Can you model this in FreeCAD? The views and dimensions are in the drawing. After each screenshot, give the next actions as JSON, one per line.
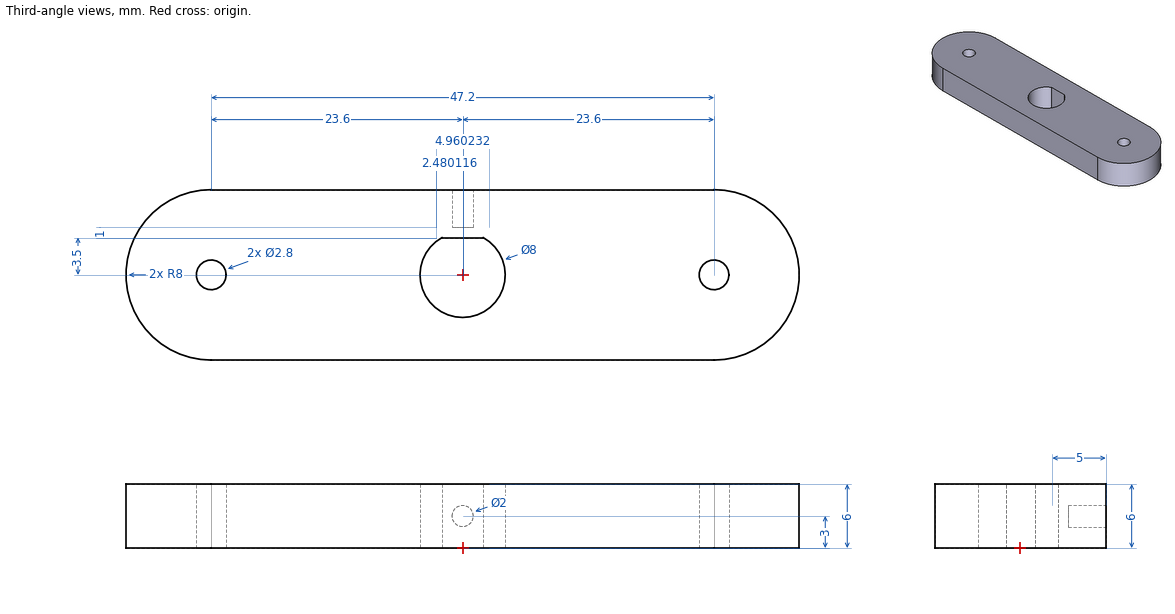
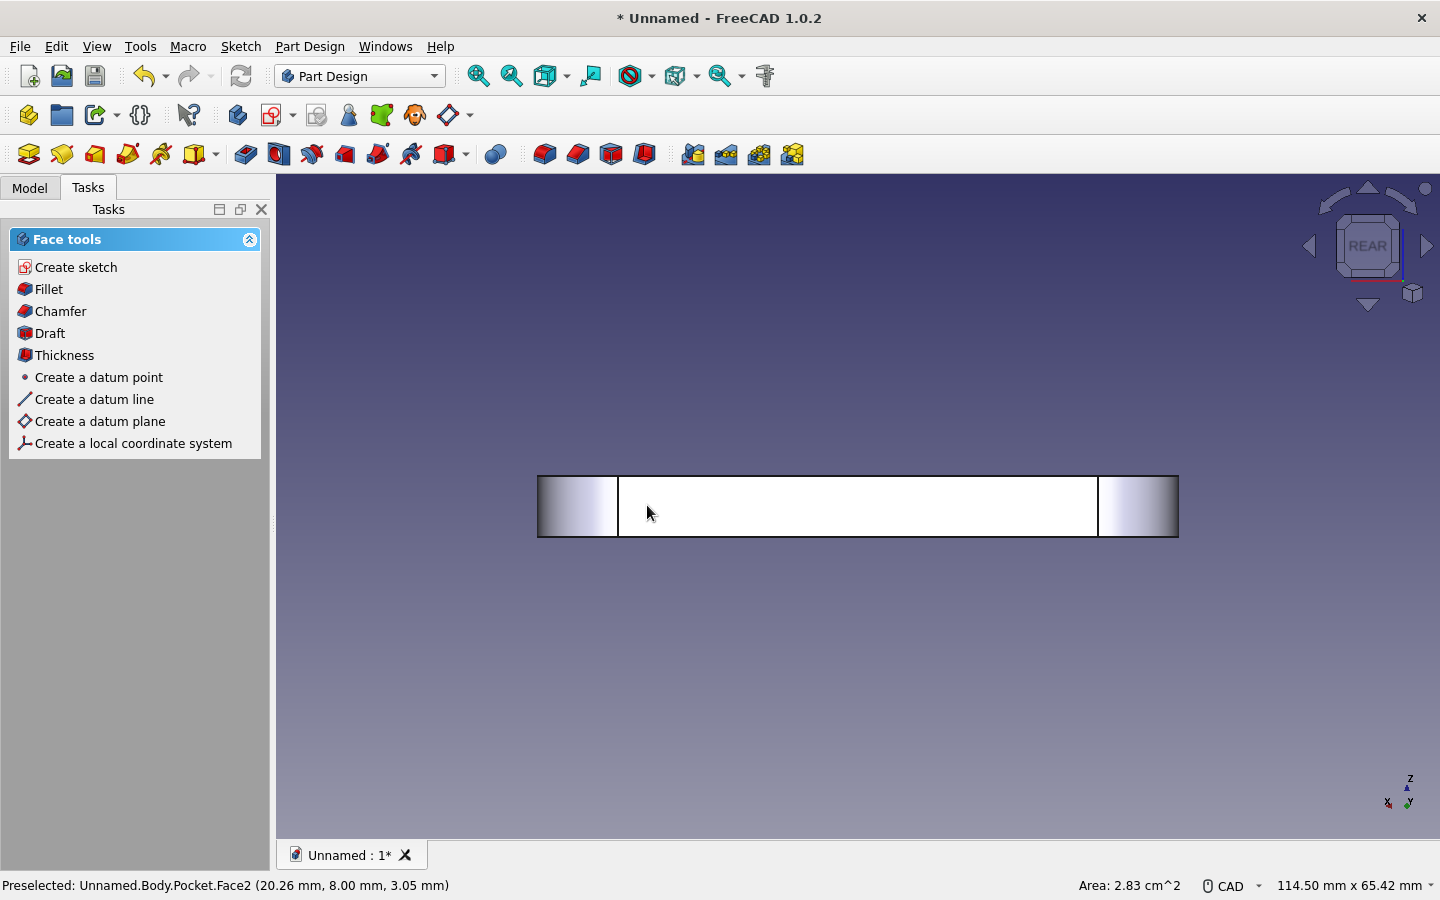
{"action": "left_click", "coordinate": [270, 116]}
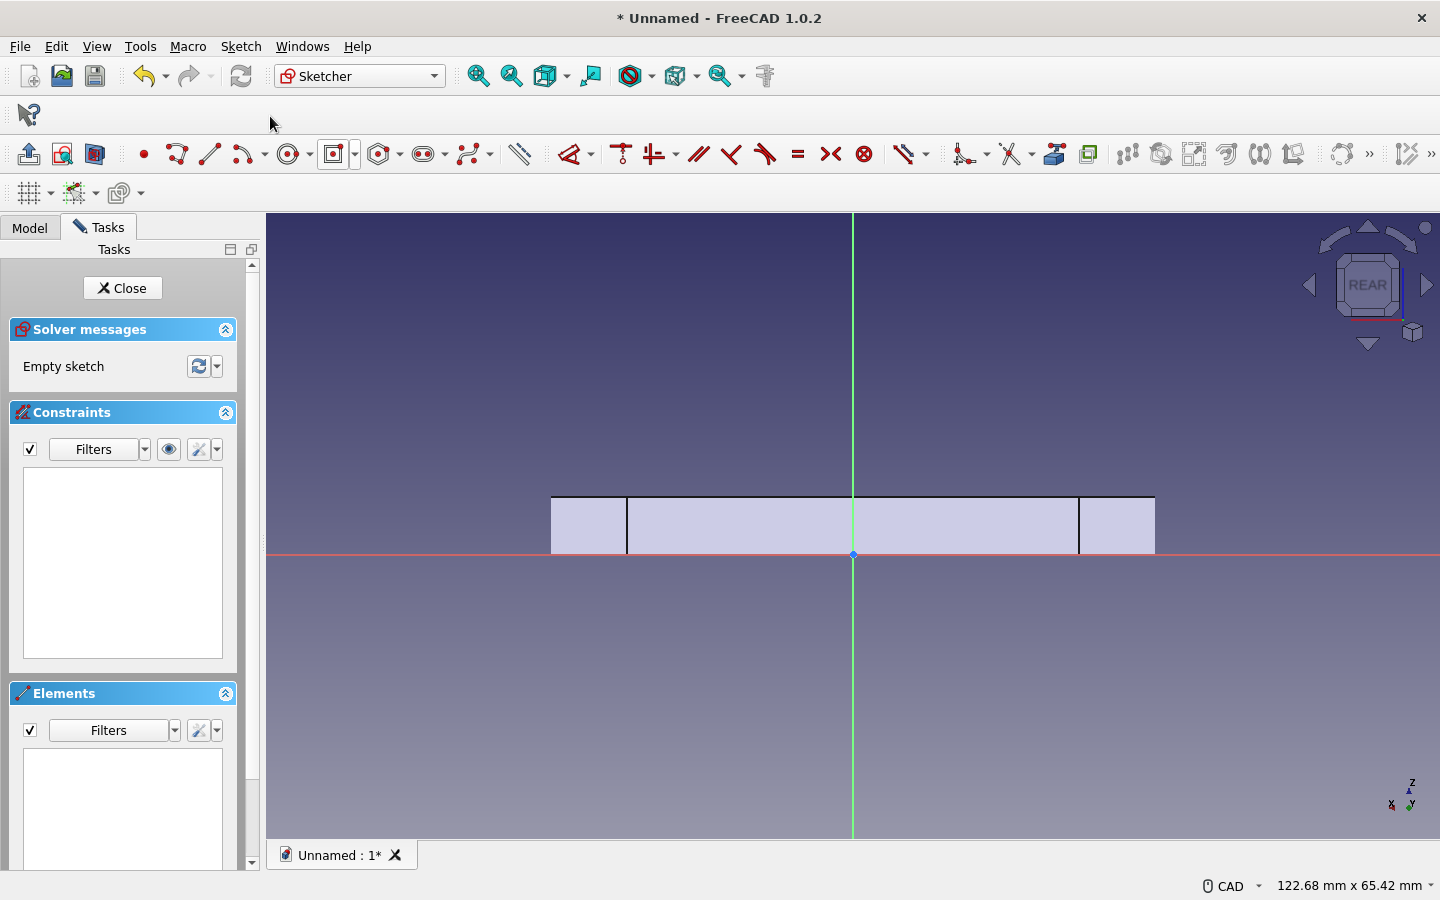
{"action": "scroll", "coordinate": [860, 537], "scroll_direction": "up", "scroll_amount": 12}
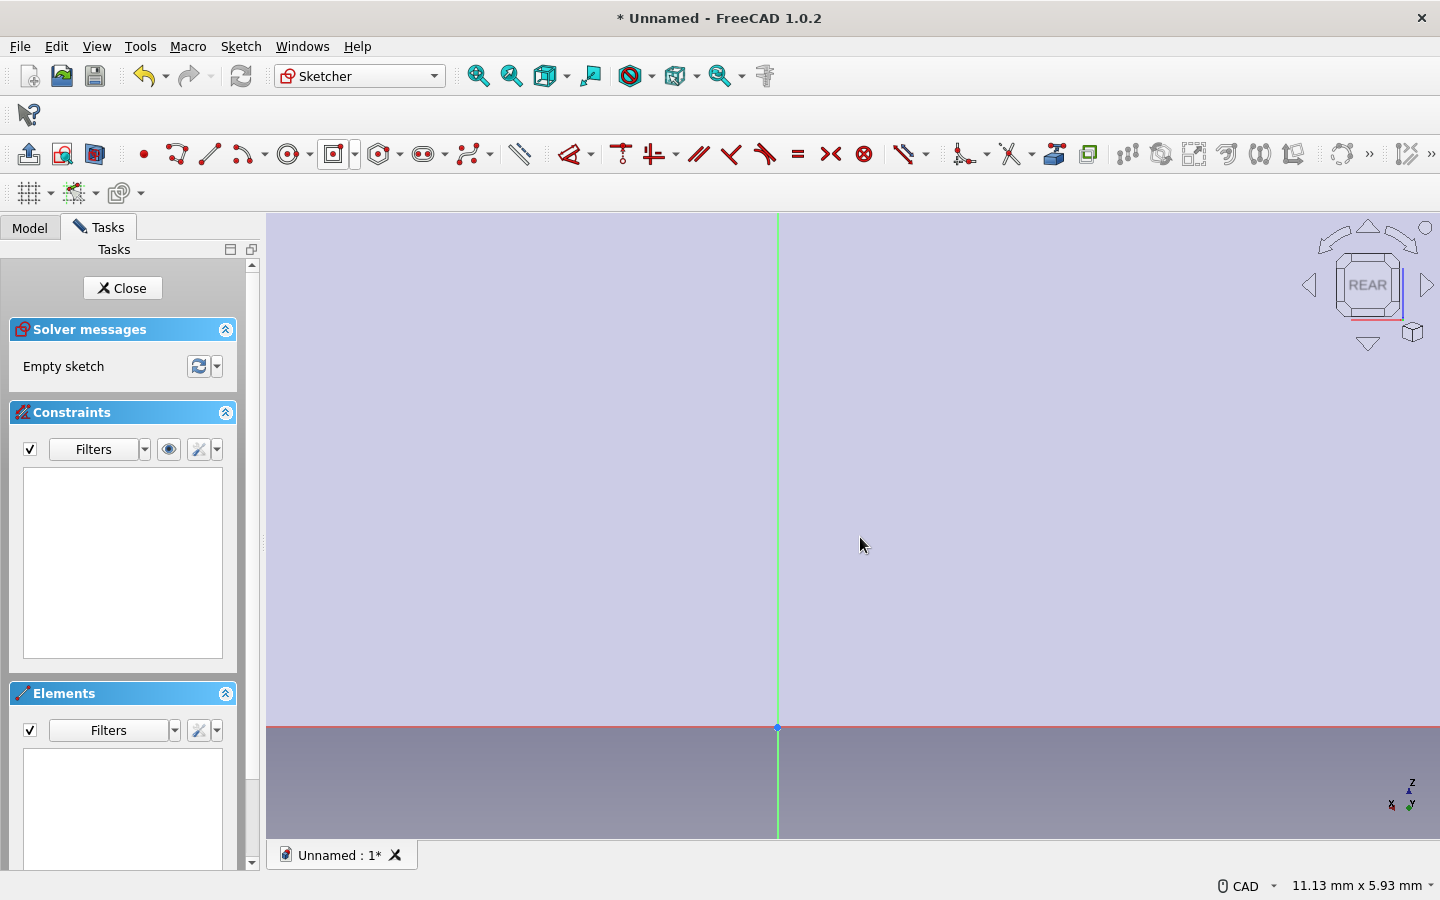
{"action": "left_click", "coordinate": [288, 154]}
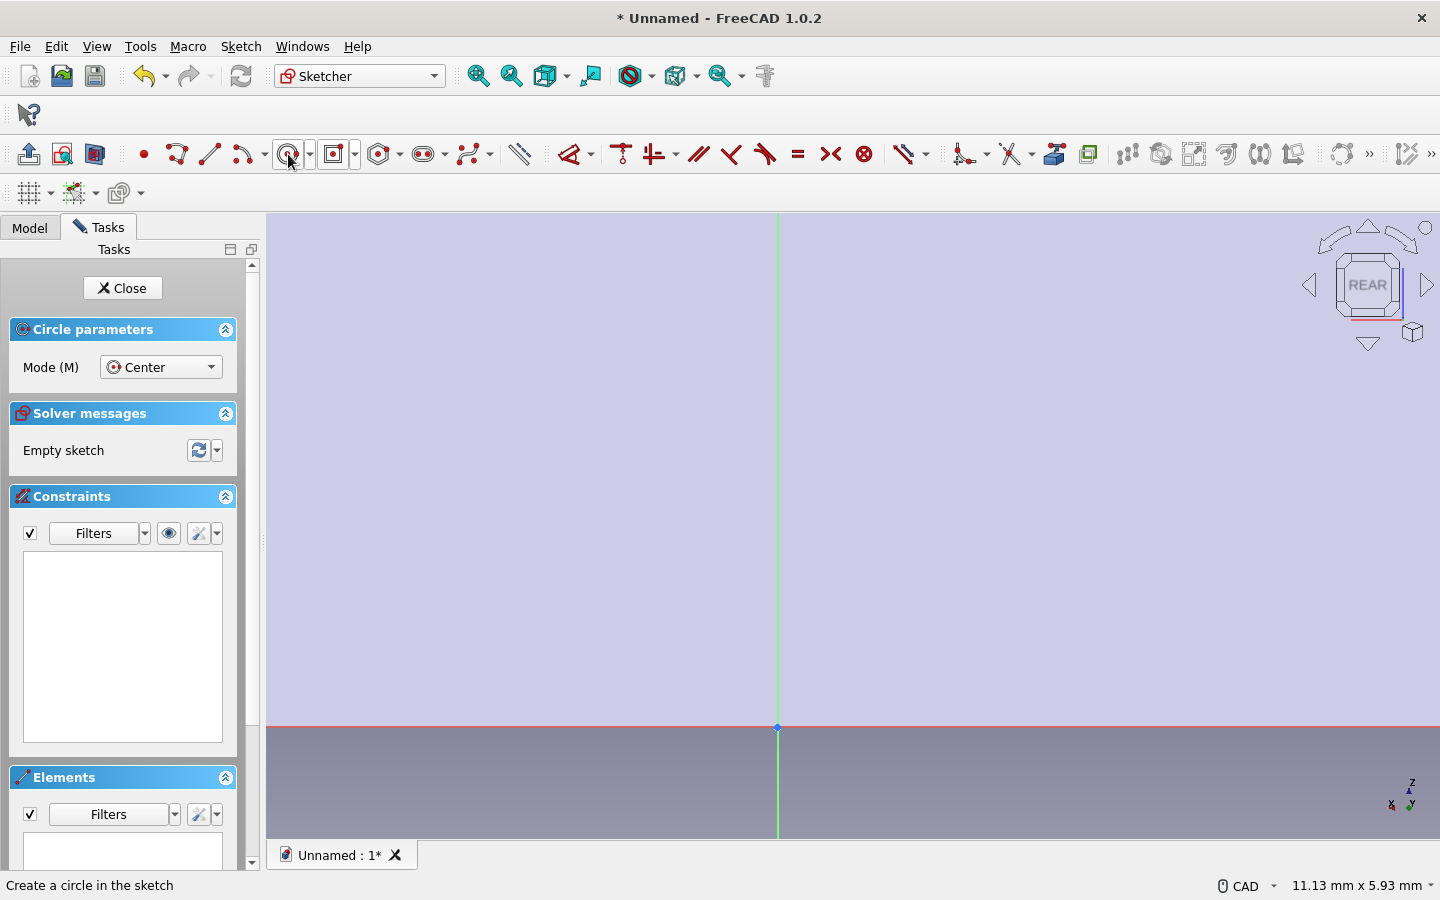
{"action": "left_click", "coordinate": [778, 411]}
{"action": "left_click", "coordinate": [852, 336]}
{"action": "key", "text": "Escape"}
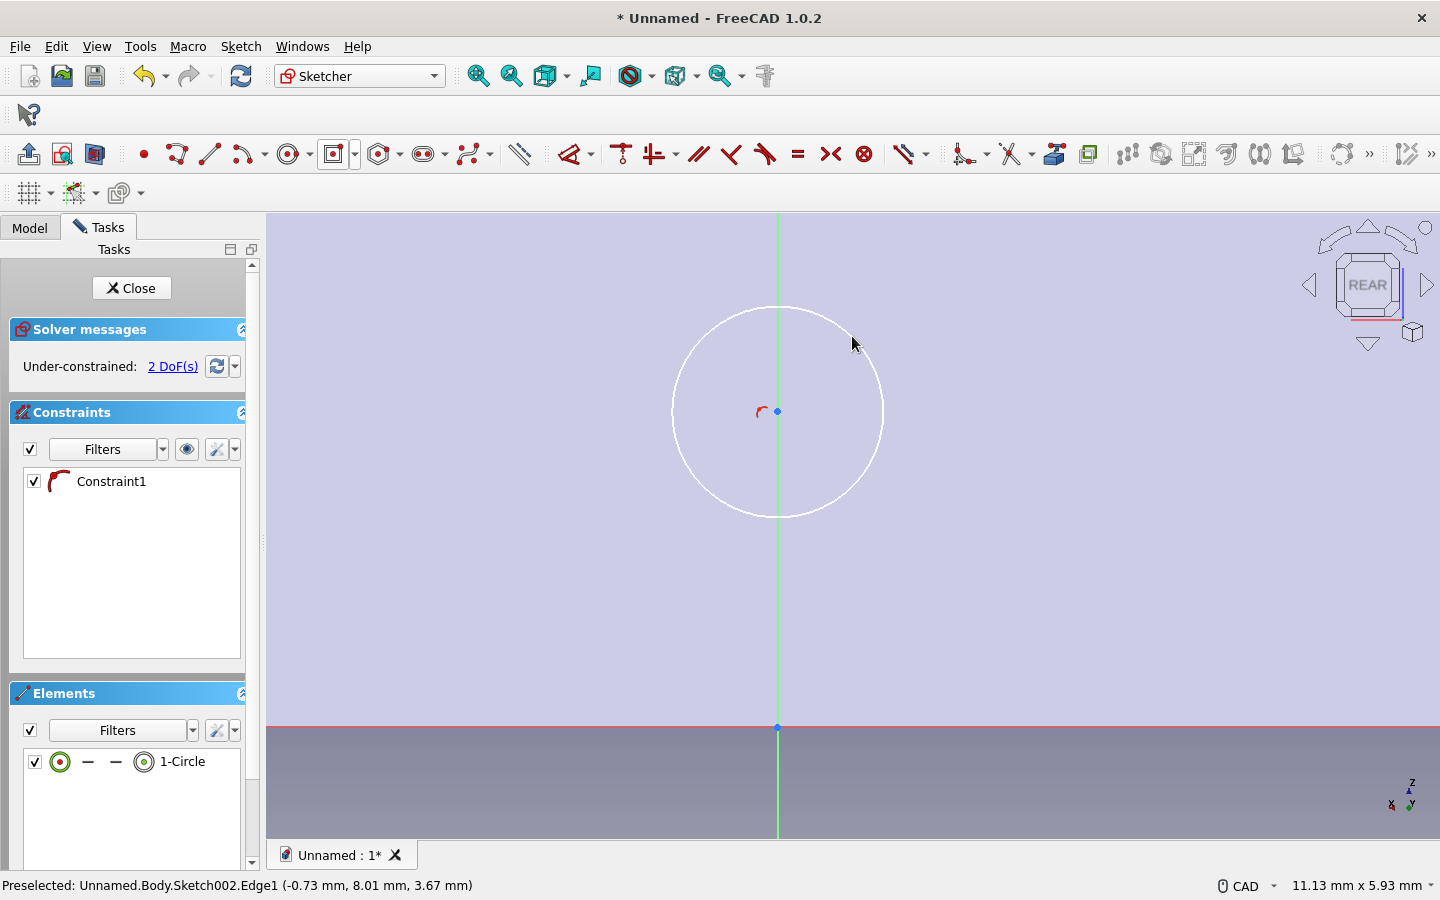
{"action": "left_click", "coordinate": [568, 154]}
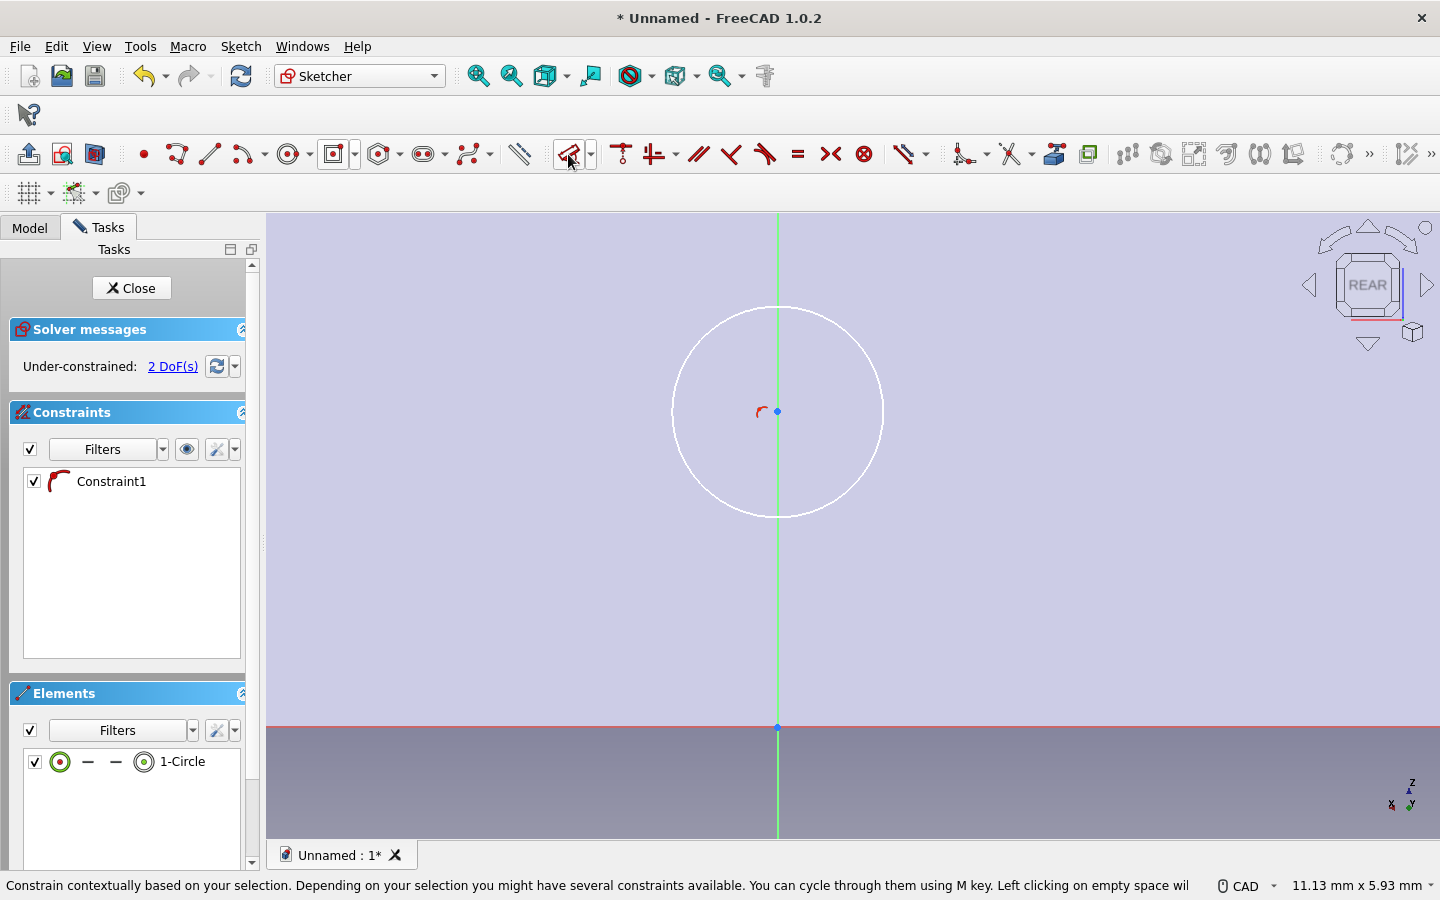
{"action": "left_click", "coordinate": [852, 337]}
{"action": "left_click", "coordinate": [875, 314]}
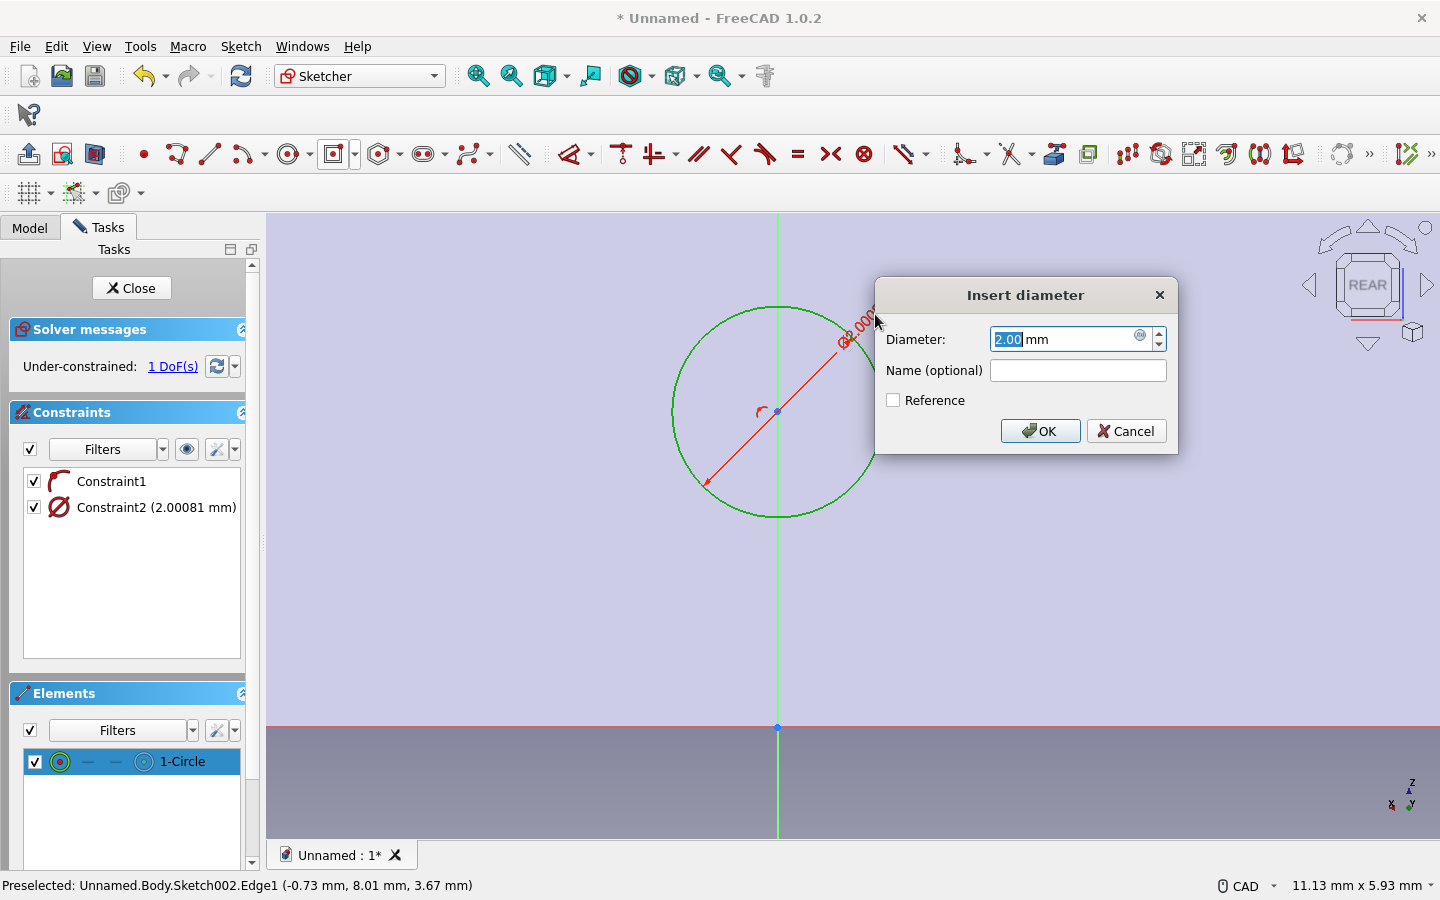
{"action": "type", "text": "2"}
{"action": "key", "text": "Return"}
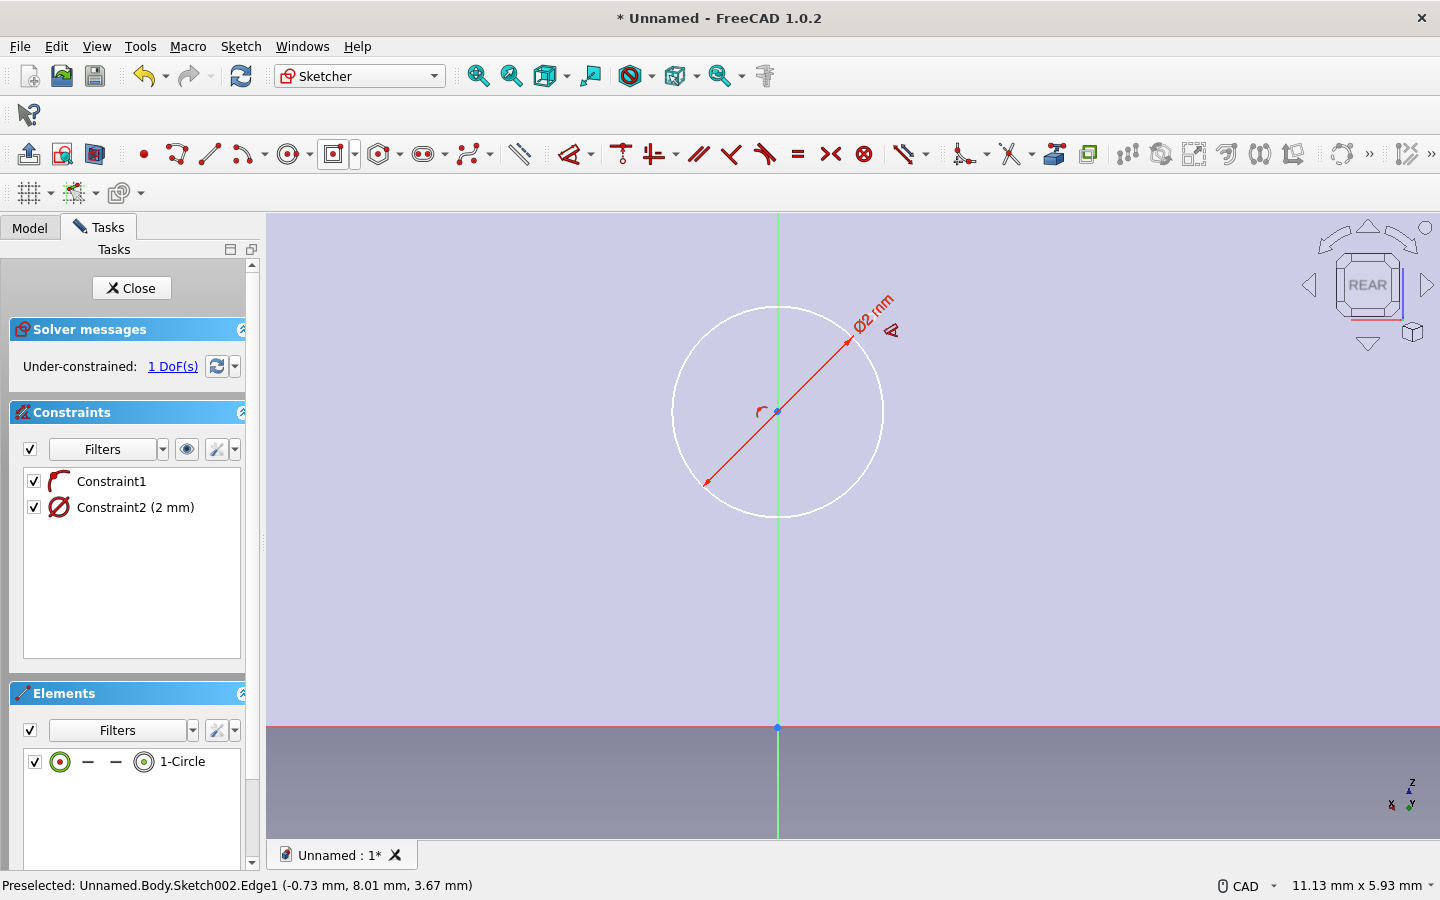
{"action": "left_click", "coordinate": [778, 412]}
{"action": "left_click", "coordinate": [812, 570]}